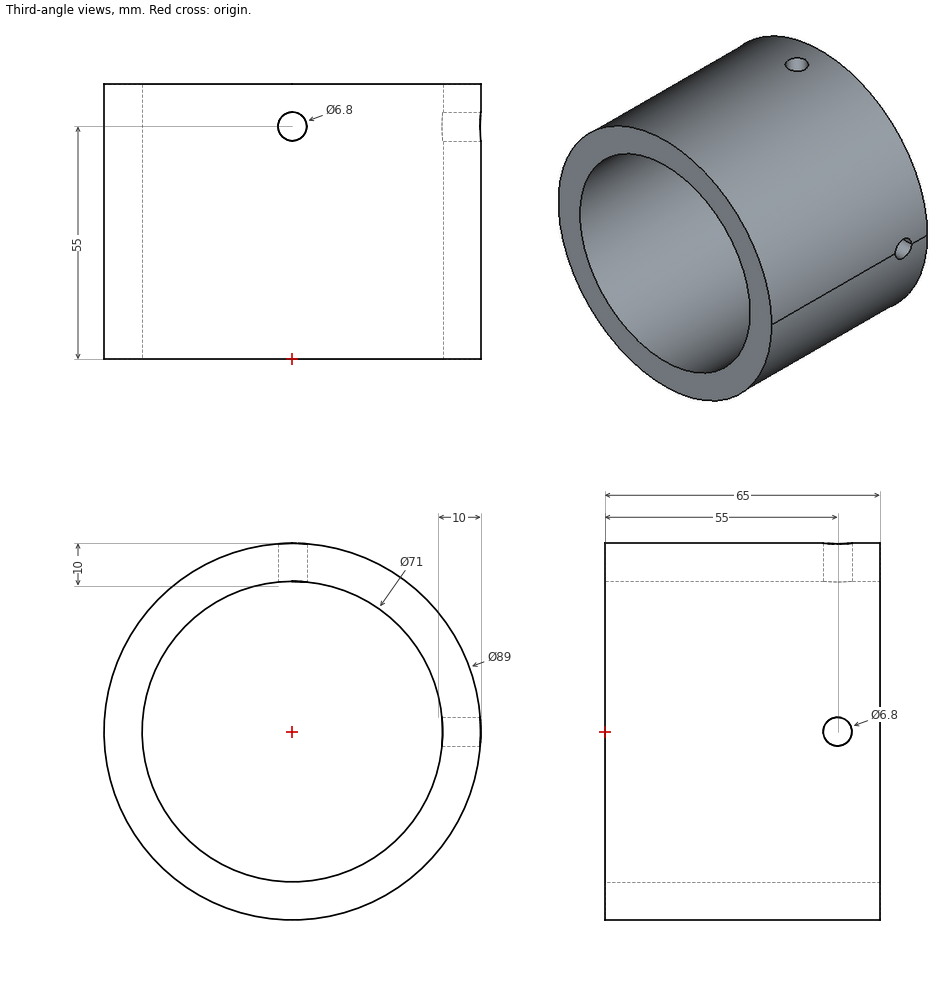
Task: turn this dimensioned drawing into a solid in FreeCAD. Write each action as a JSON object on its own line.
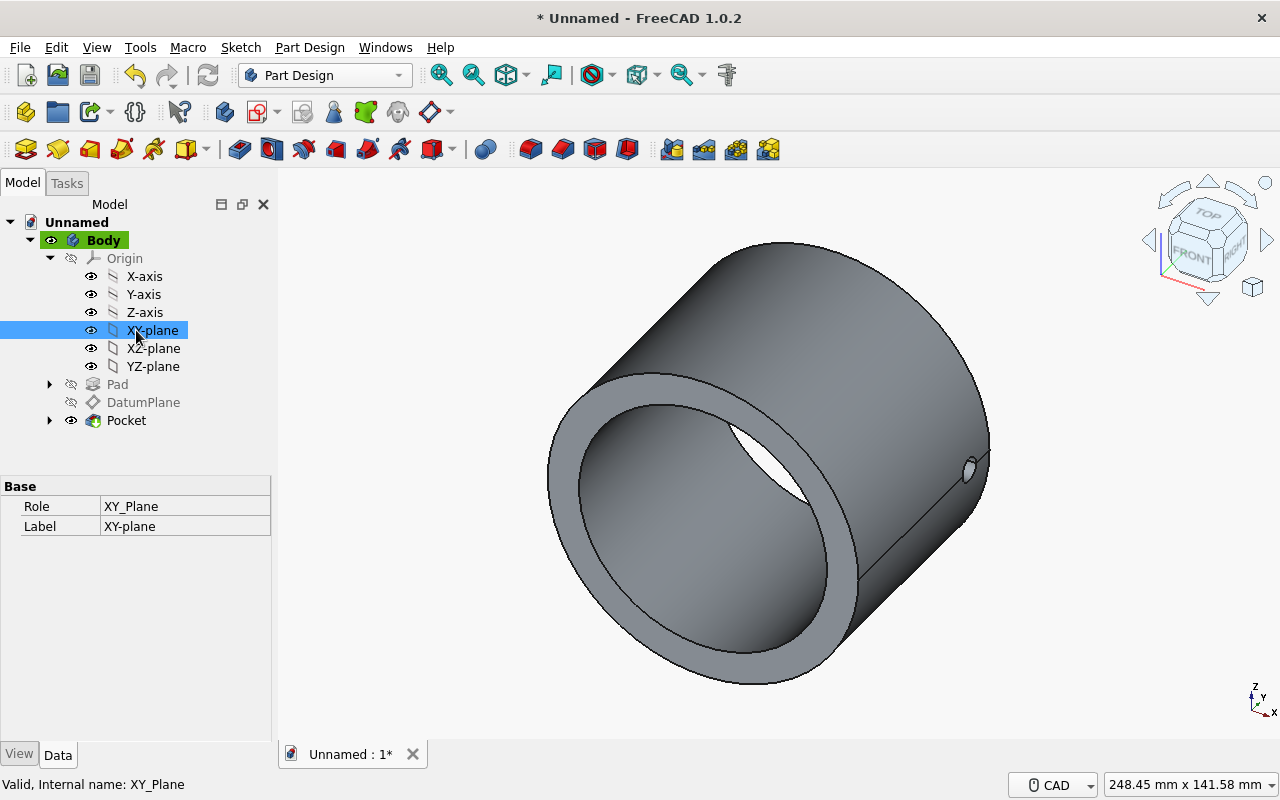
{"action": "left_click", "coordinate": [430, 112]}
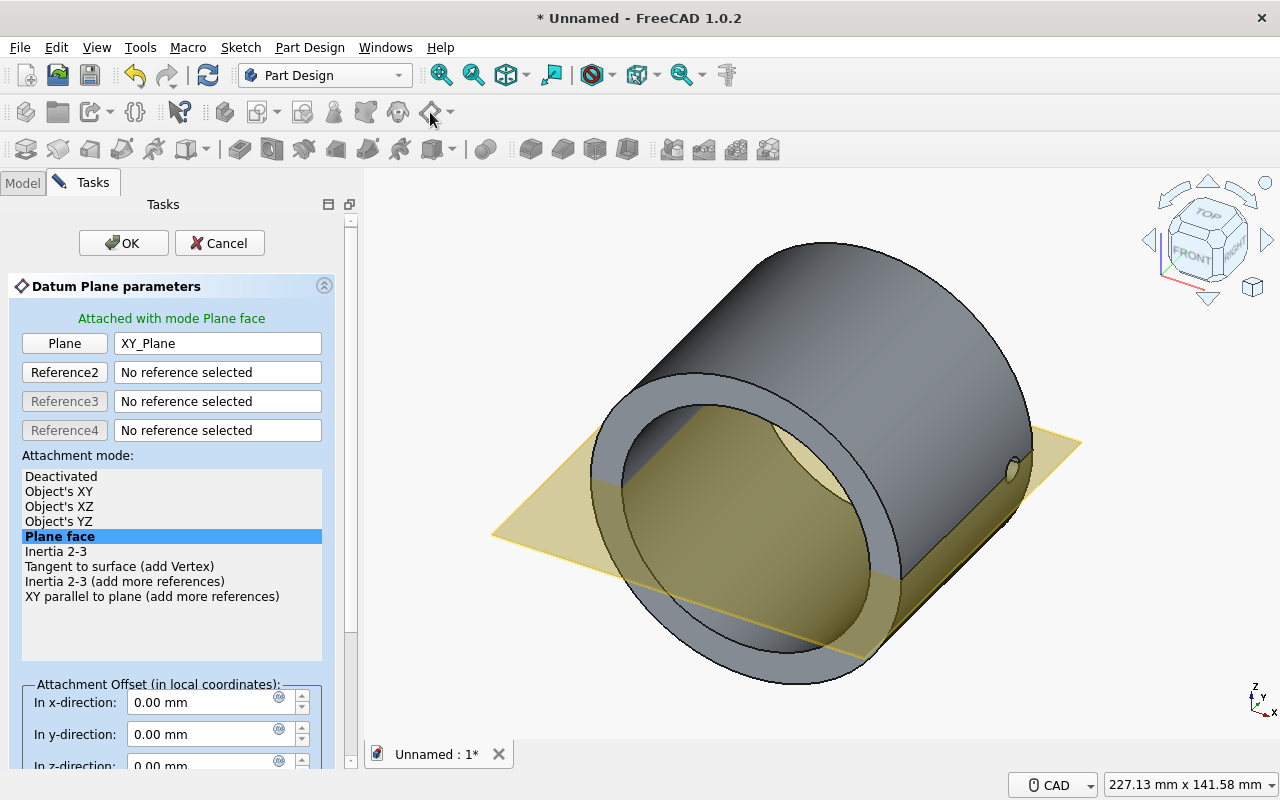
{"action": "scroll", "coordinate": [351, 491], "scroll_direction": "down", "scroll_amount": 2}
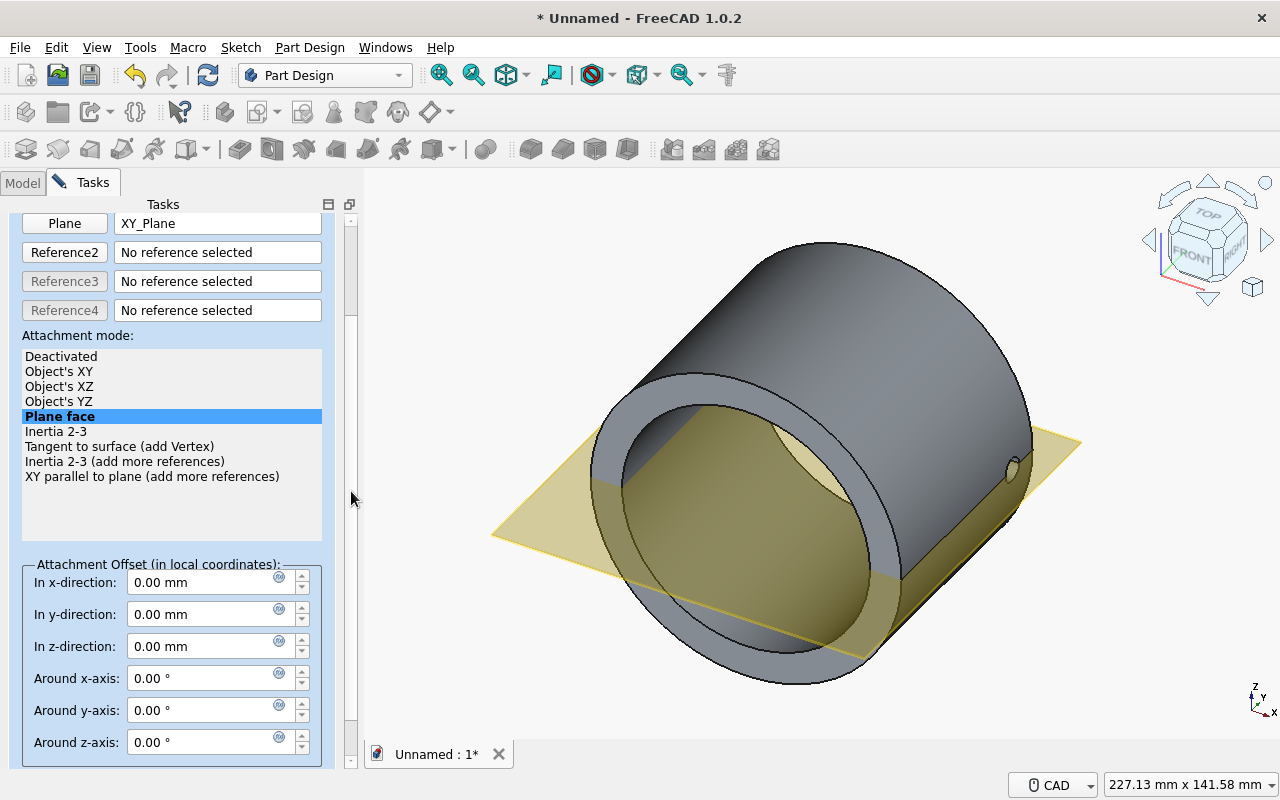
{"action": "triple_click", "coordinate": [210, 646]}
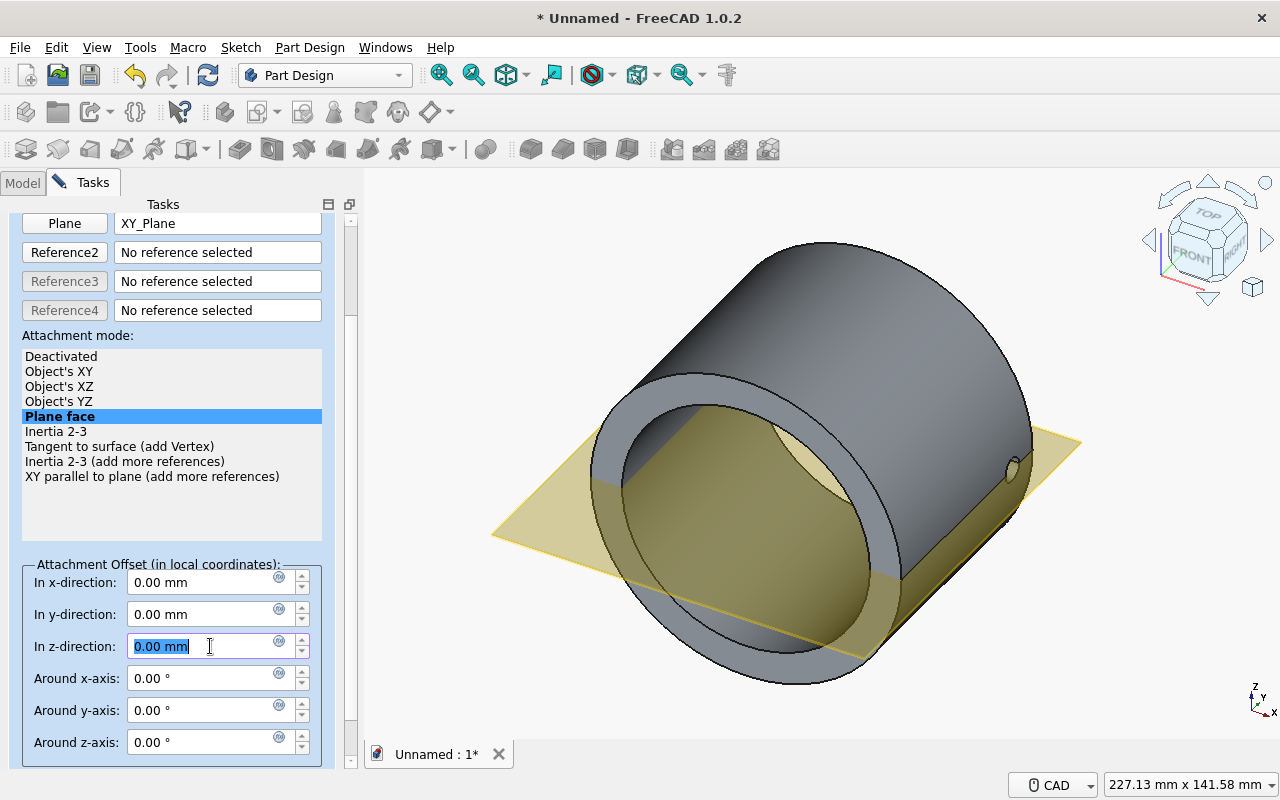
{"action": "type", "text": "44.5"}
{"action": "key", "text": "Tab"}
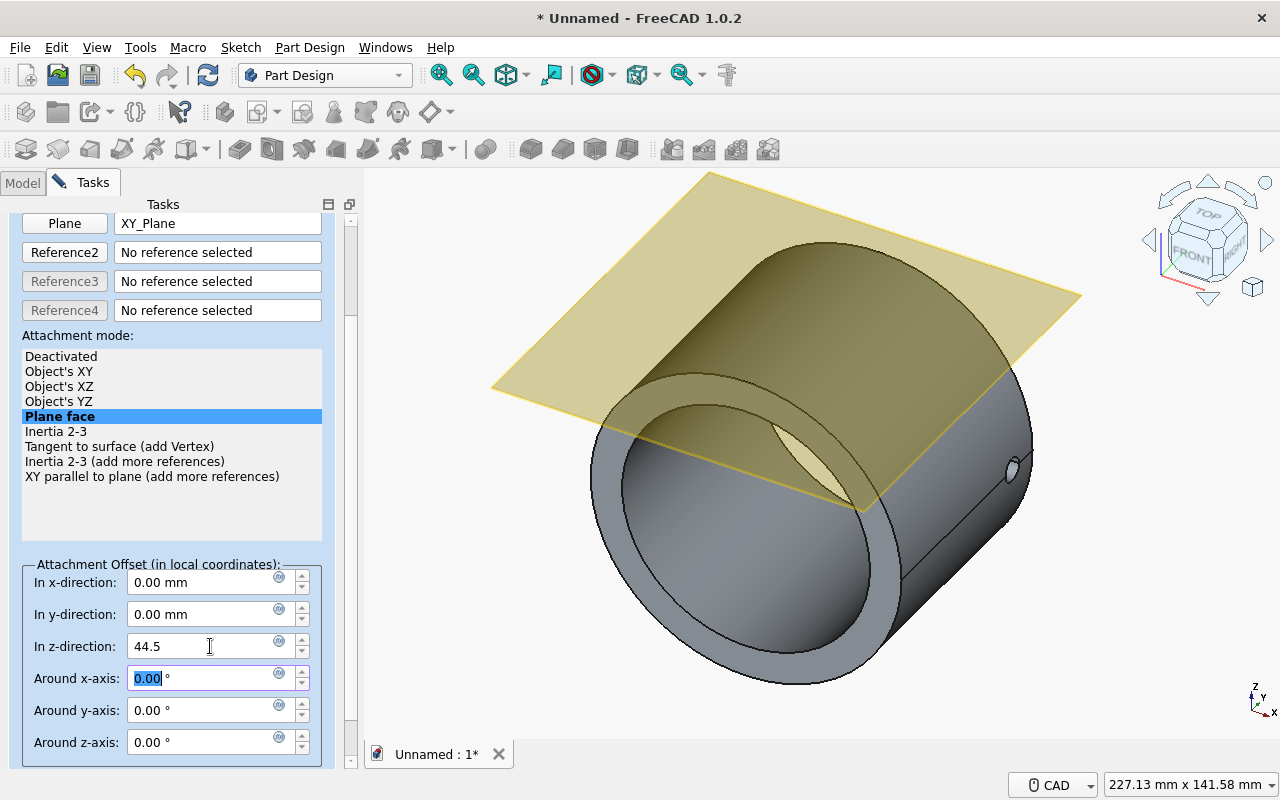
{"action": "scroll", "coordinate": [351, 491], "scroll_direction": "up", "scroll_amount": 3}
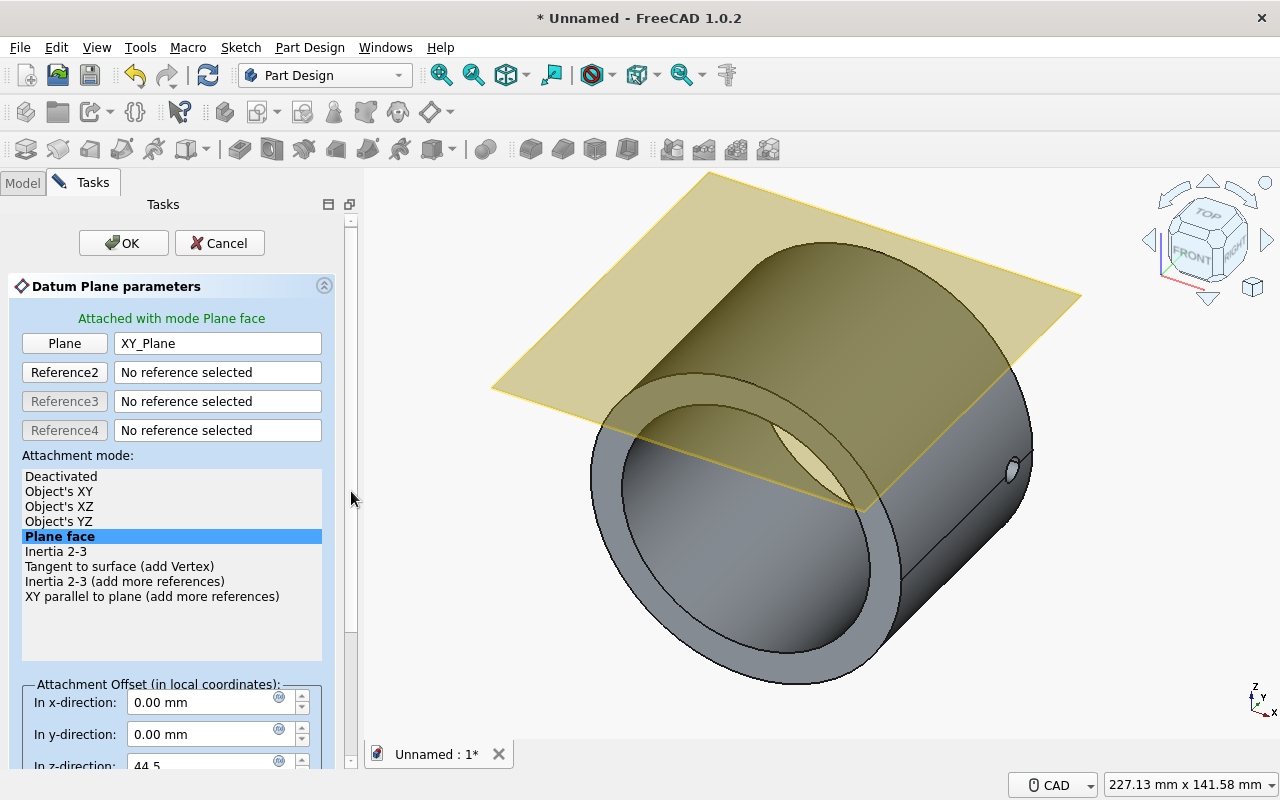
{"action": "left_click", "coordinate": [124, 243]}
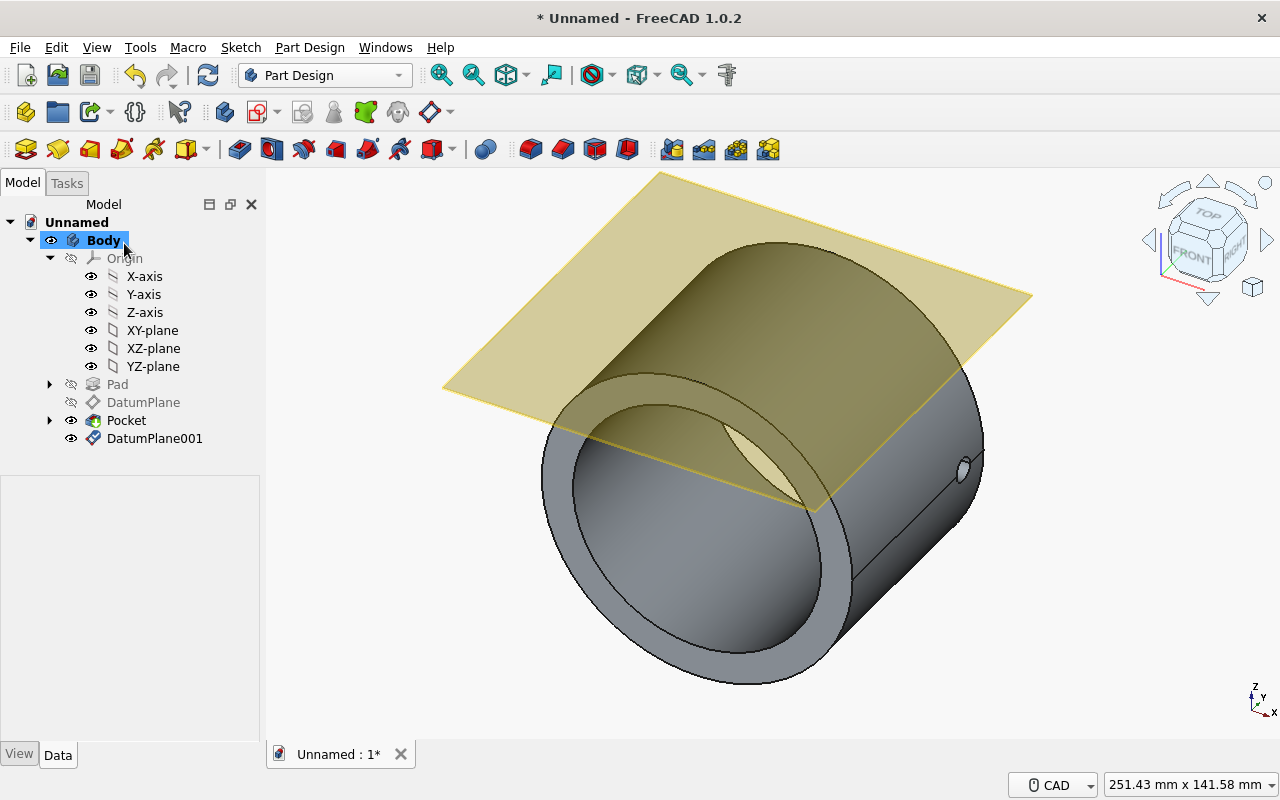
{"action": "left_click", "coordinate": [116, 438]}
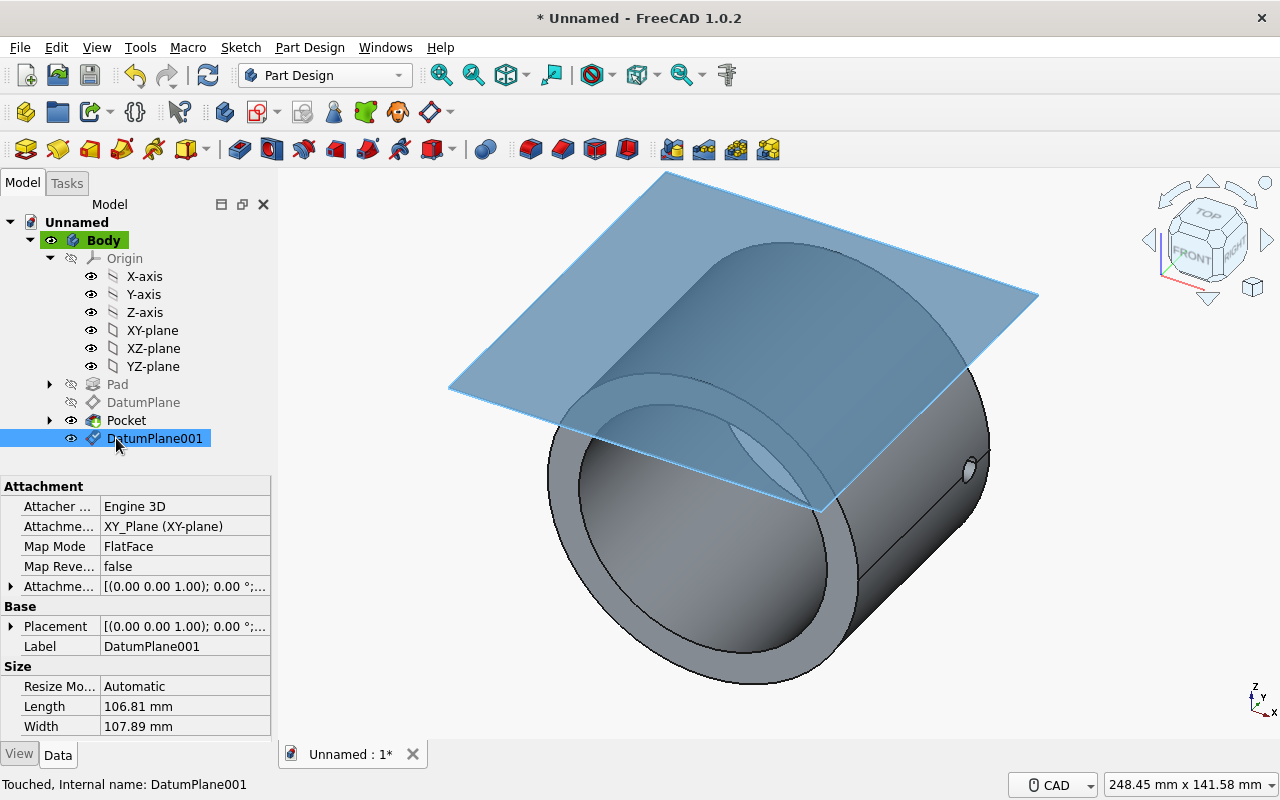
{"action": "left_click", "coordinate": [258, 112]}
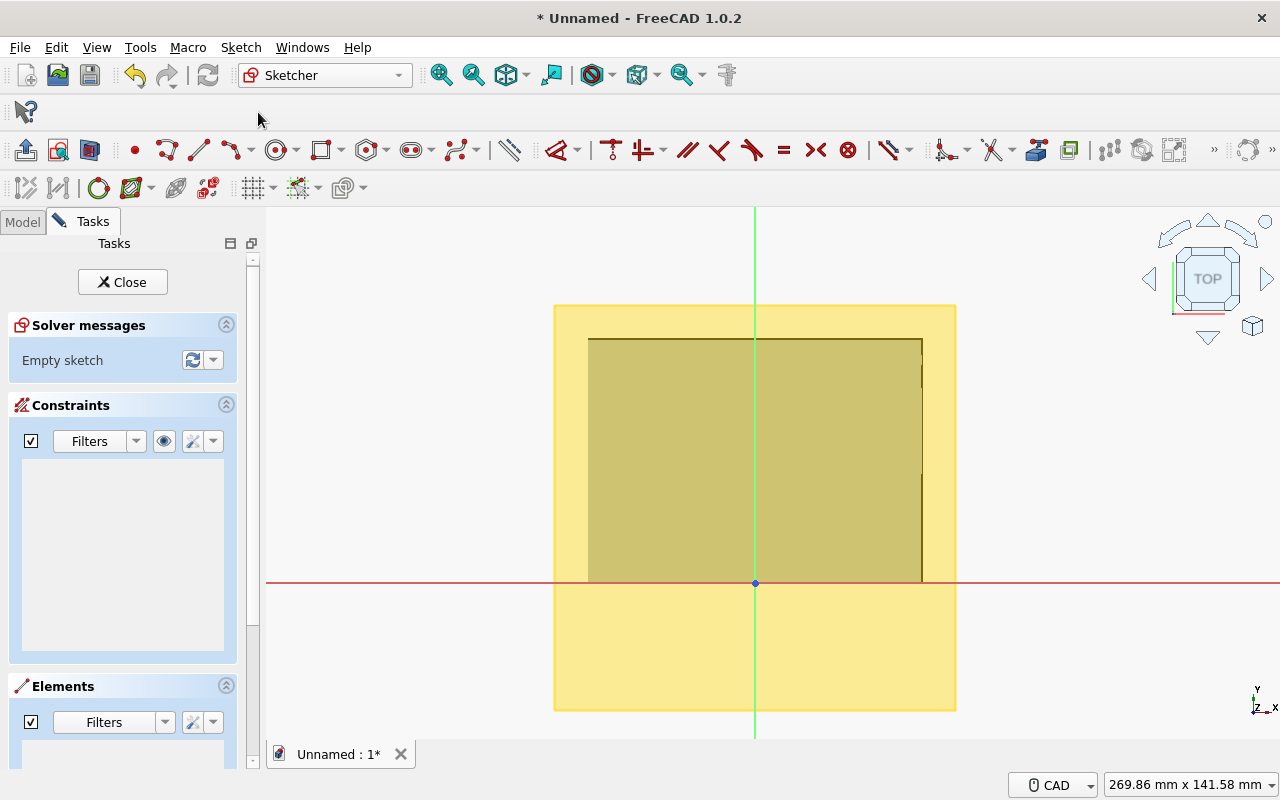
{"action": "scroll", "coordinate": [759, 369], "scroll_direction": "up", "scroll_amount": 13}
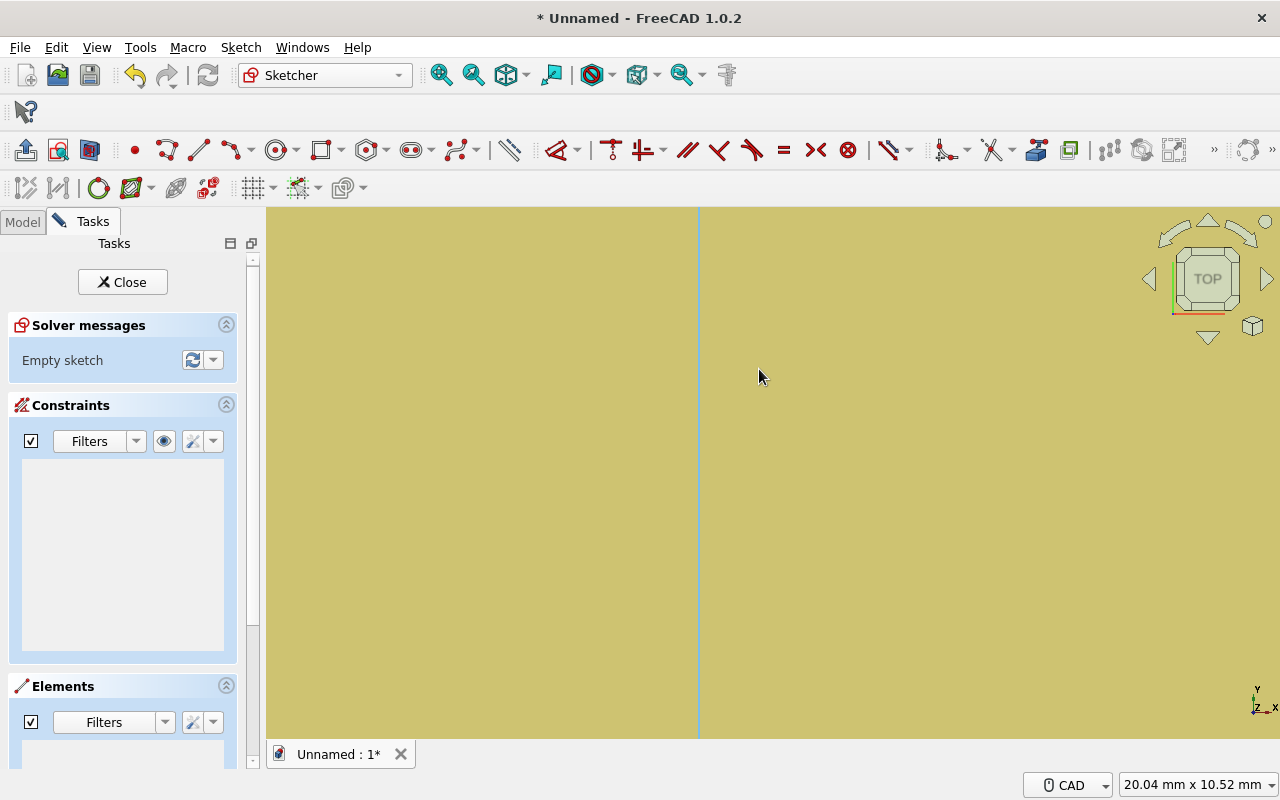
{"action": "key", "text": "g c"}